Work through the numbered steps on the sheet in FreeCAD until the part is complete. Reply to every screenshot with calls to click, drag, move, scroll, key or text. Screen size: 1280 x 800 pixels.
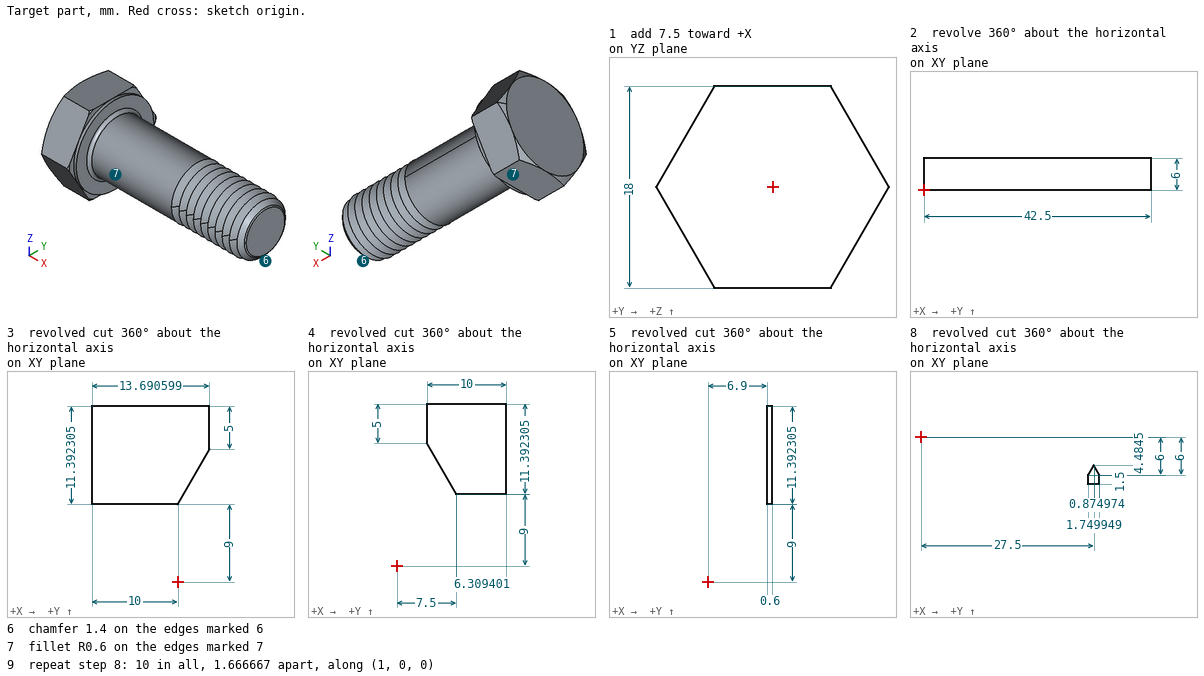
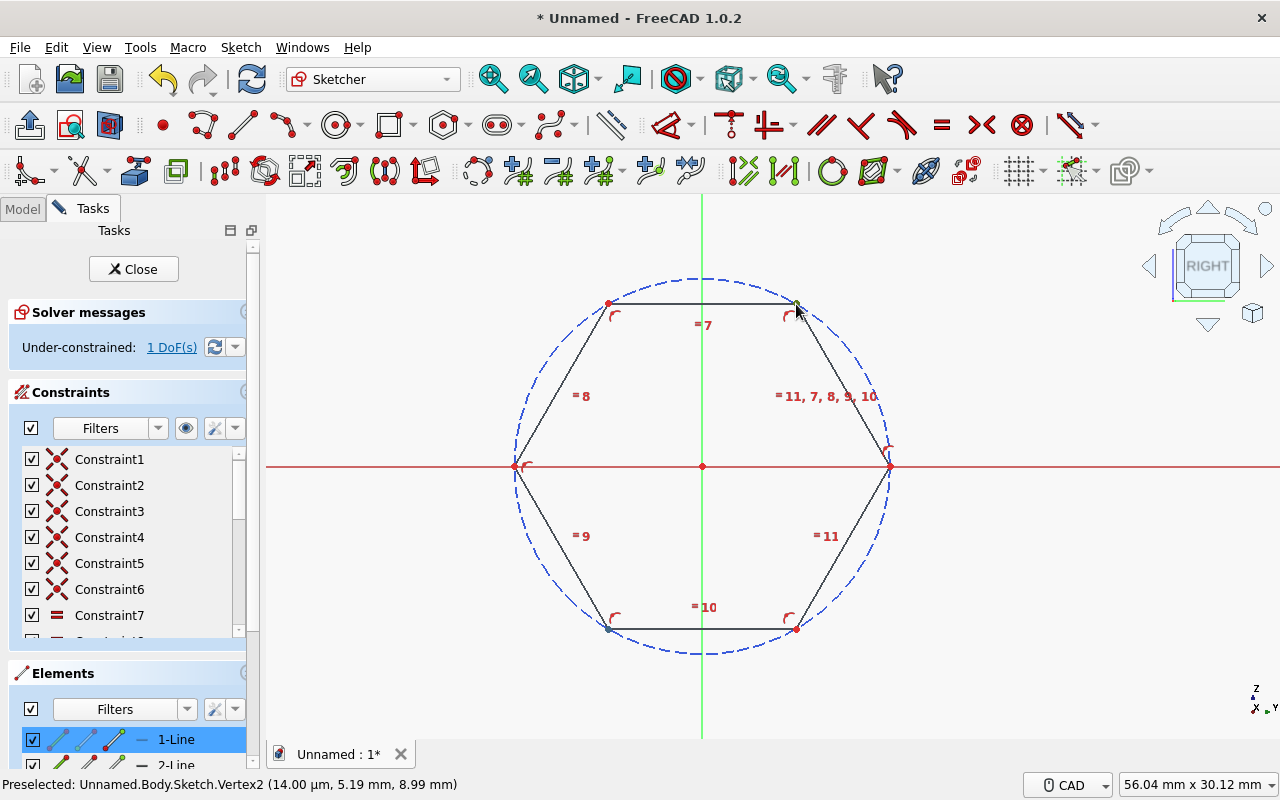
key(i)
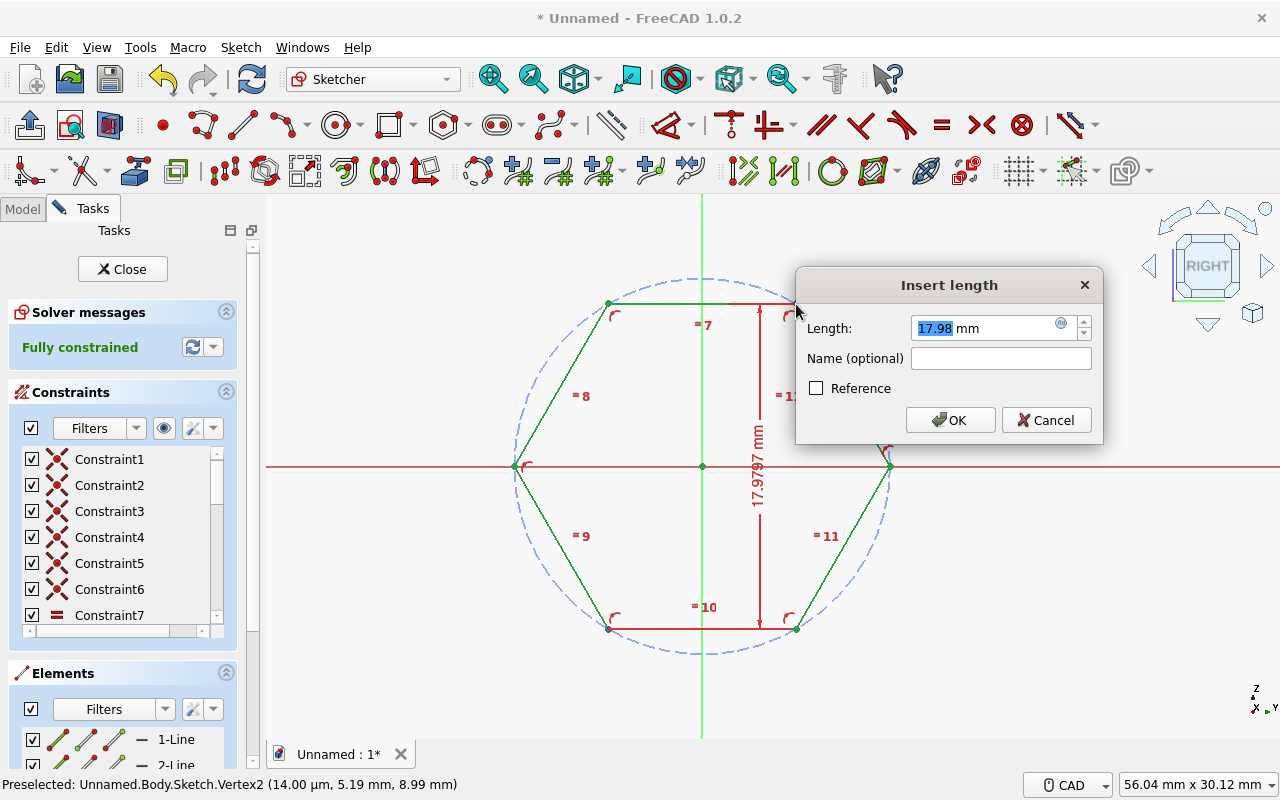
text(18)
key(Return)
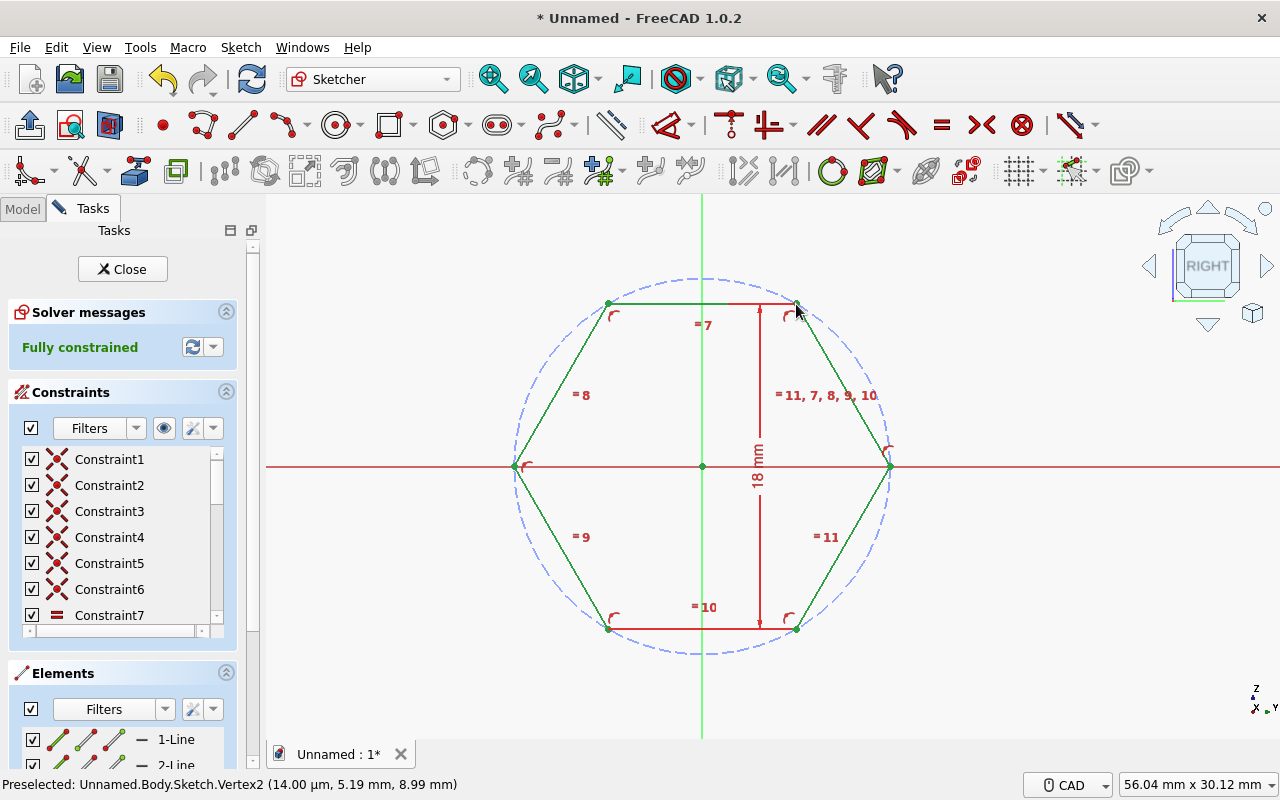
click(123, 269)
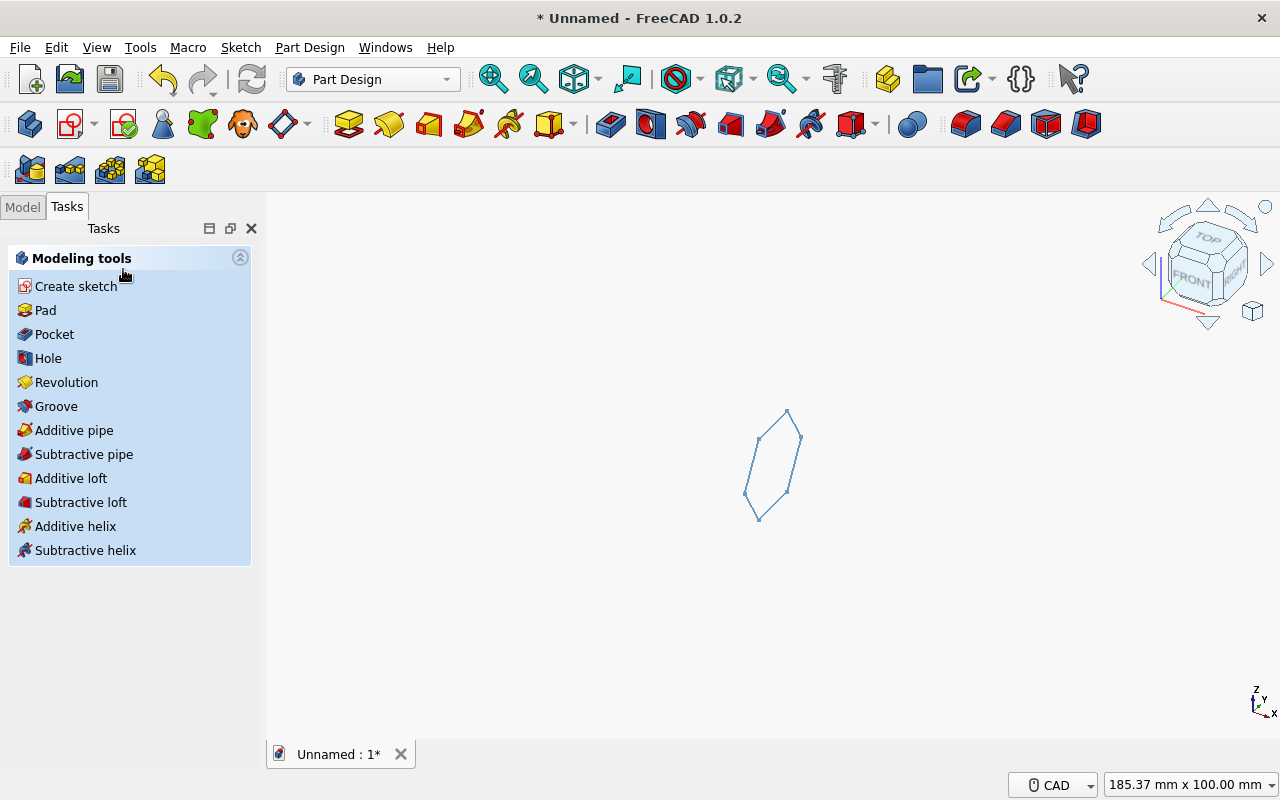
click(350, 124)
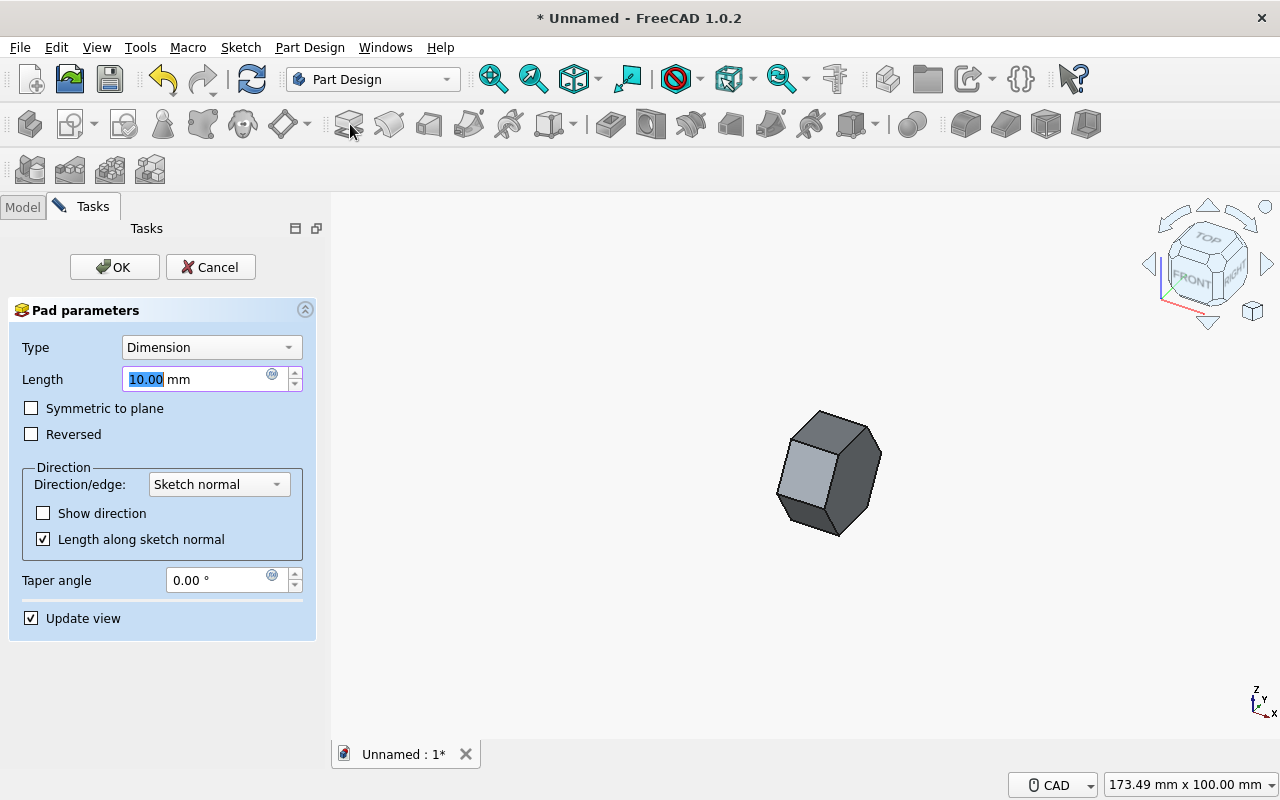
text(7.5)
key(Tab)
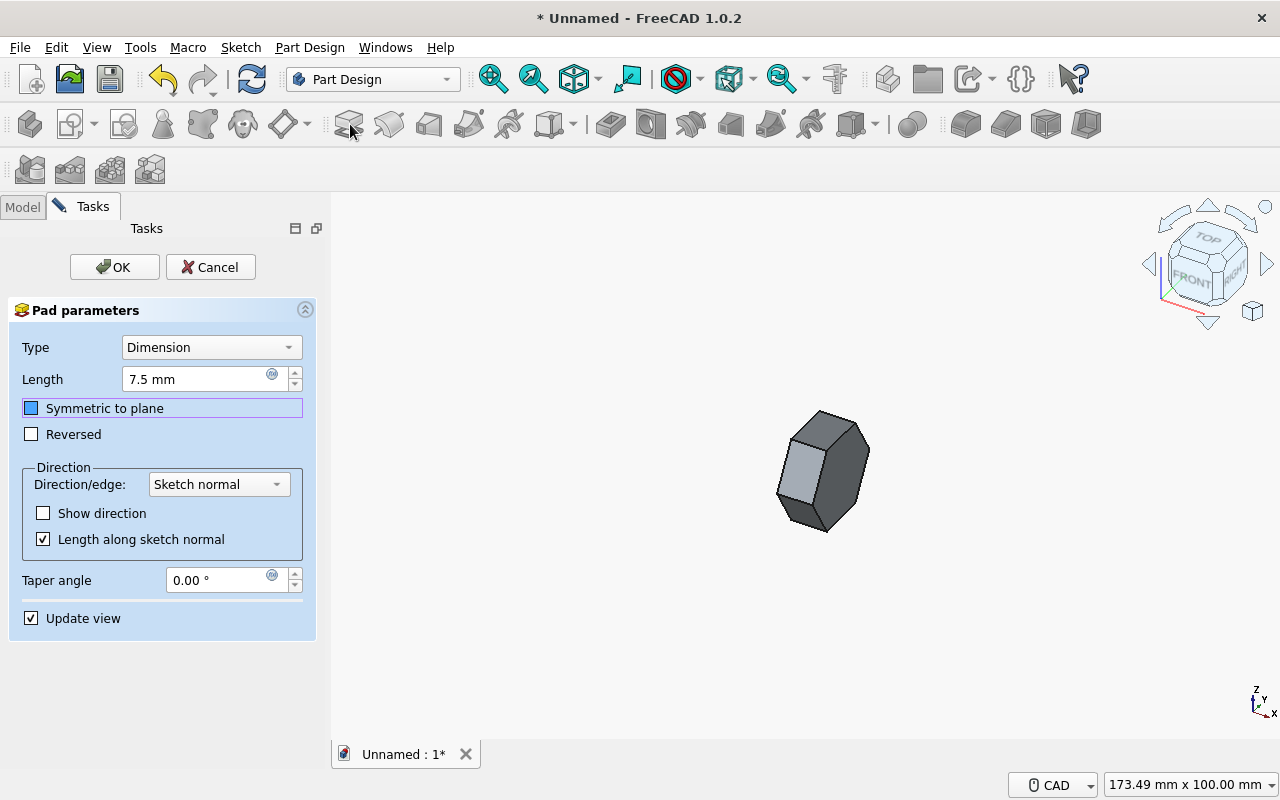
click(115, 267)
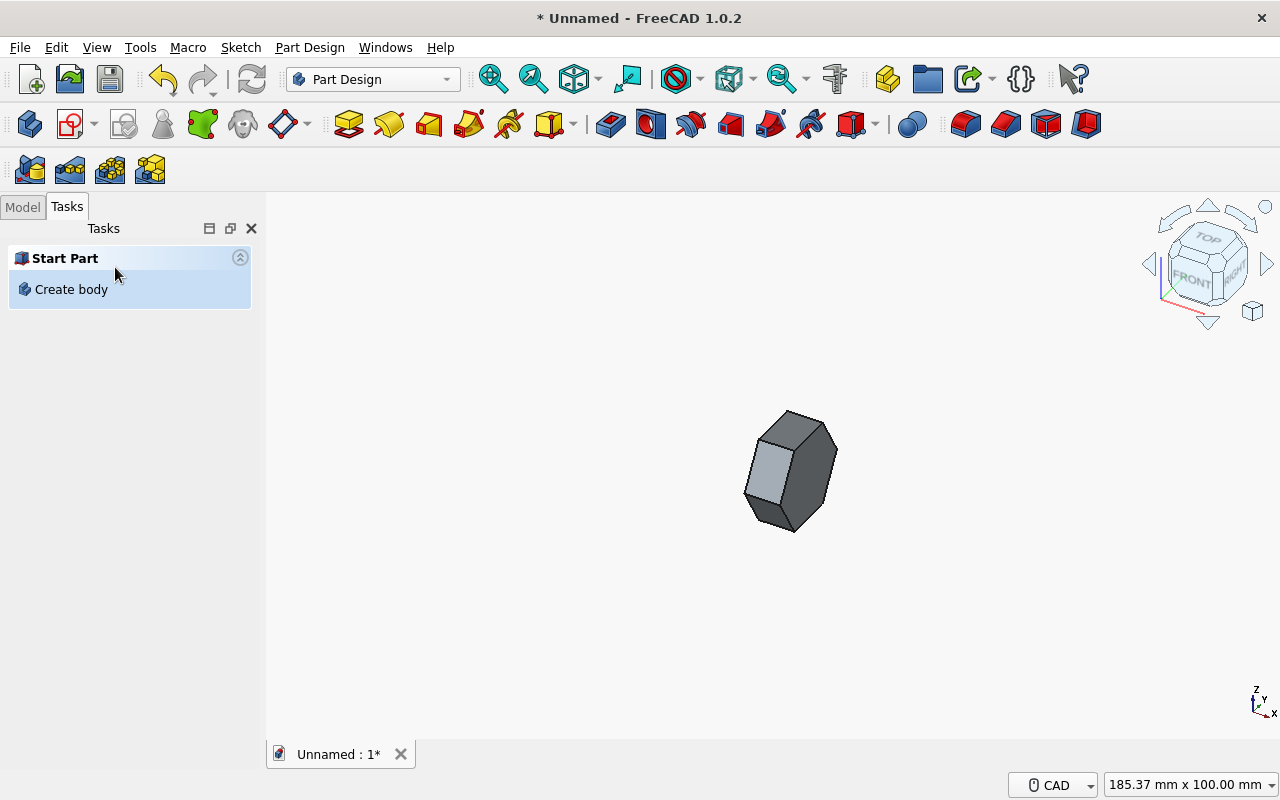
click(494, 80)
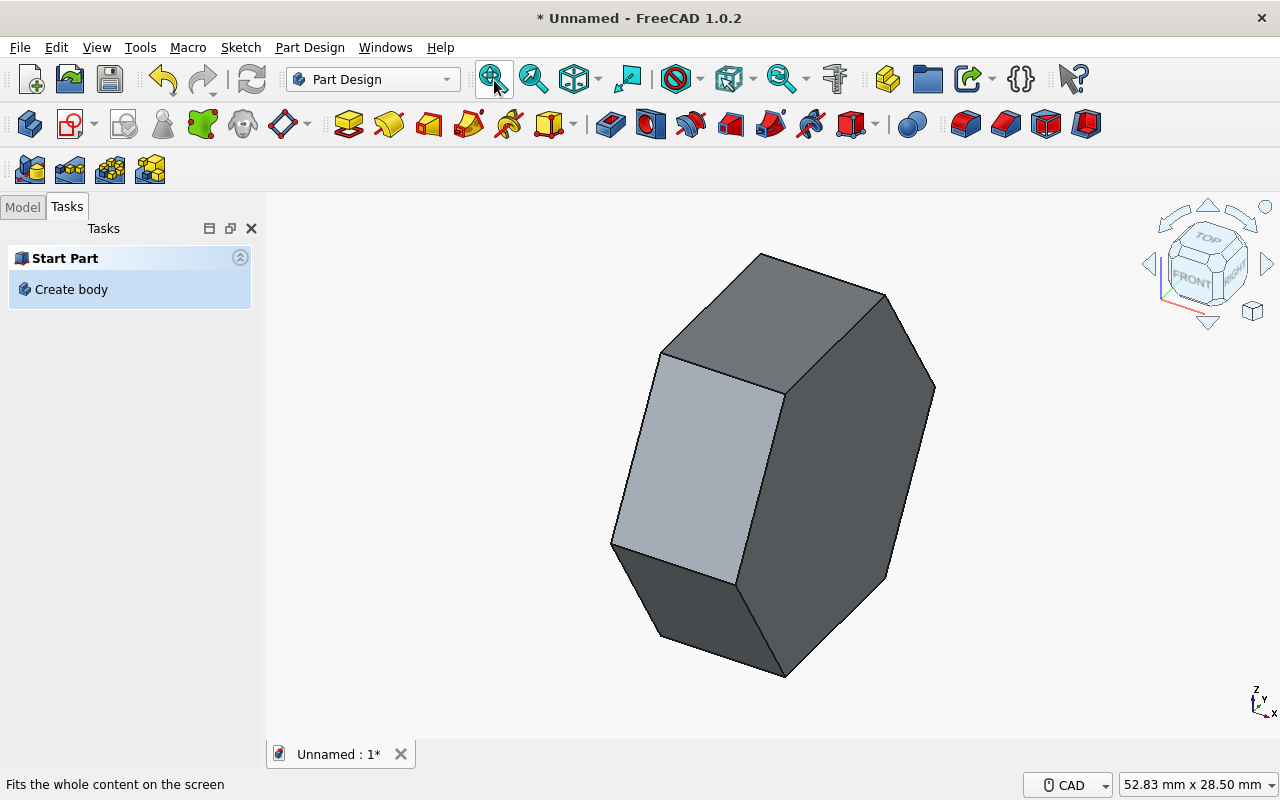
click(70, 124)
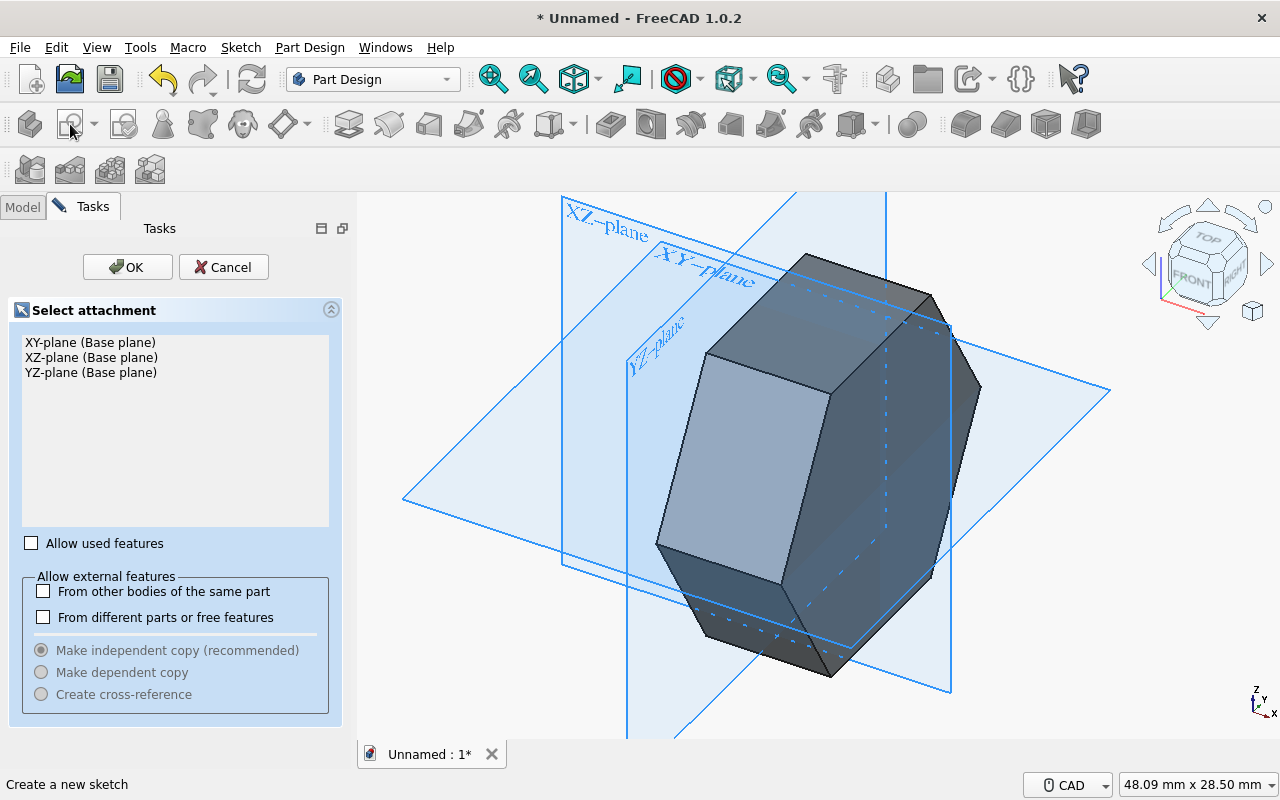
click(82, 342)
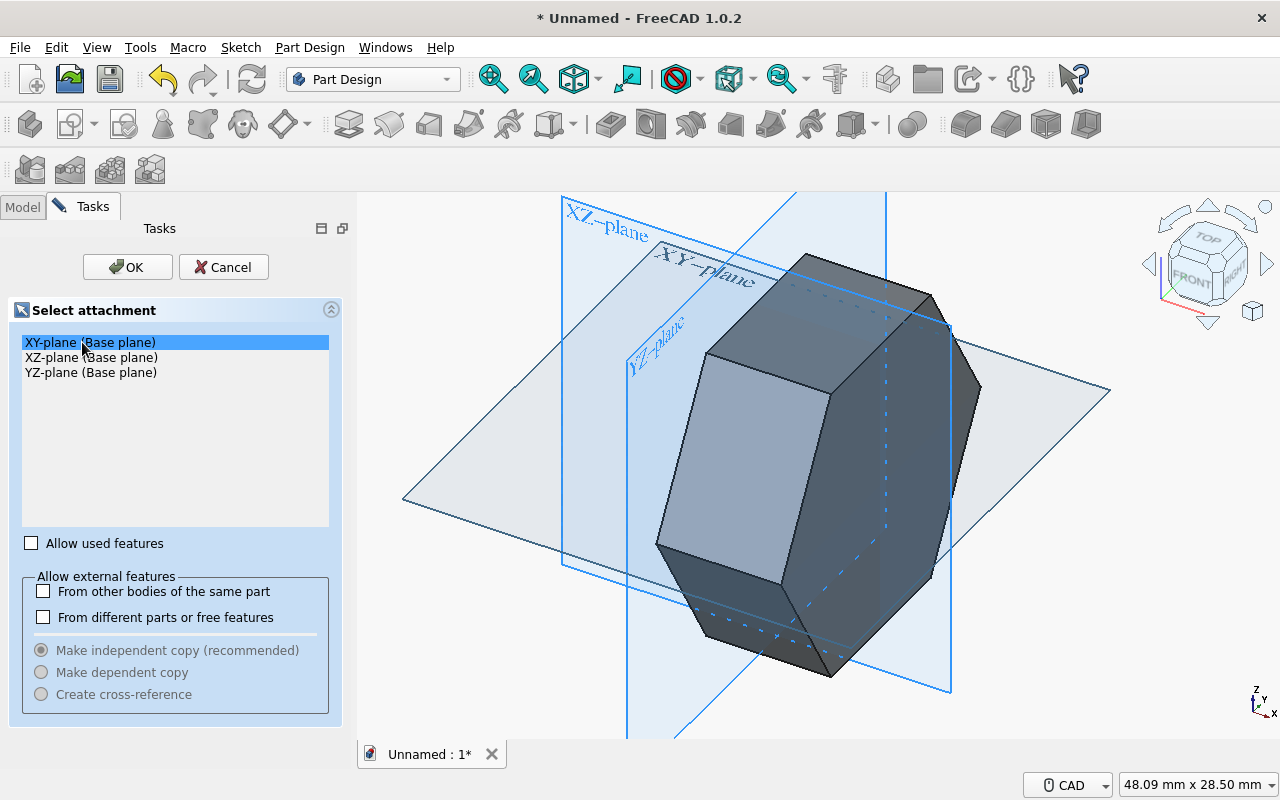
click(128, 267)